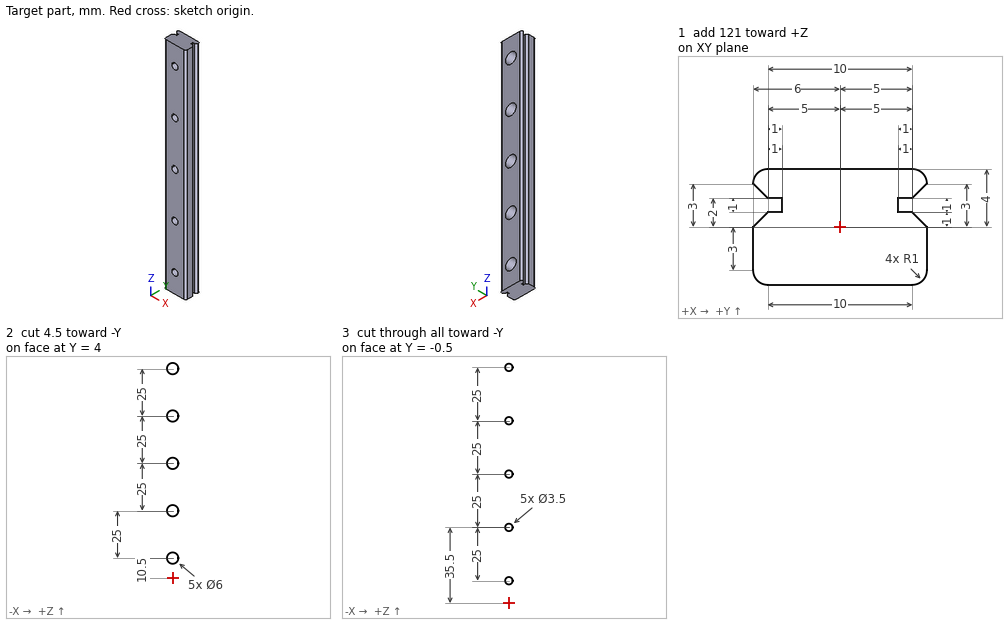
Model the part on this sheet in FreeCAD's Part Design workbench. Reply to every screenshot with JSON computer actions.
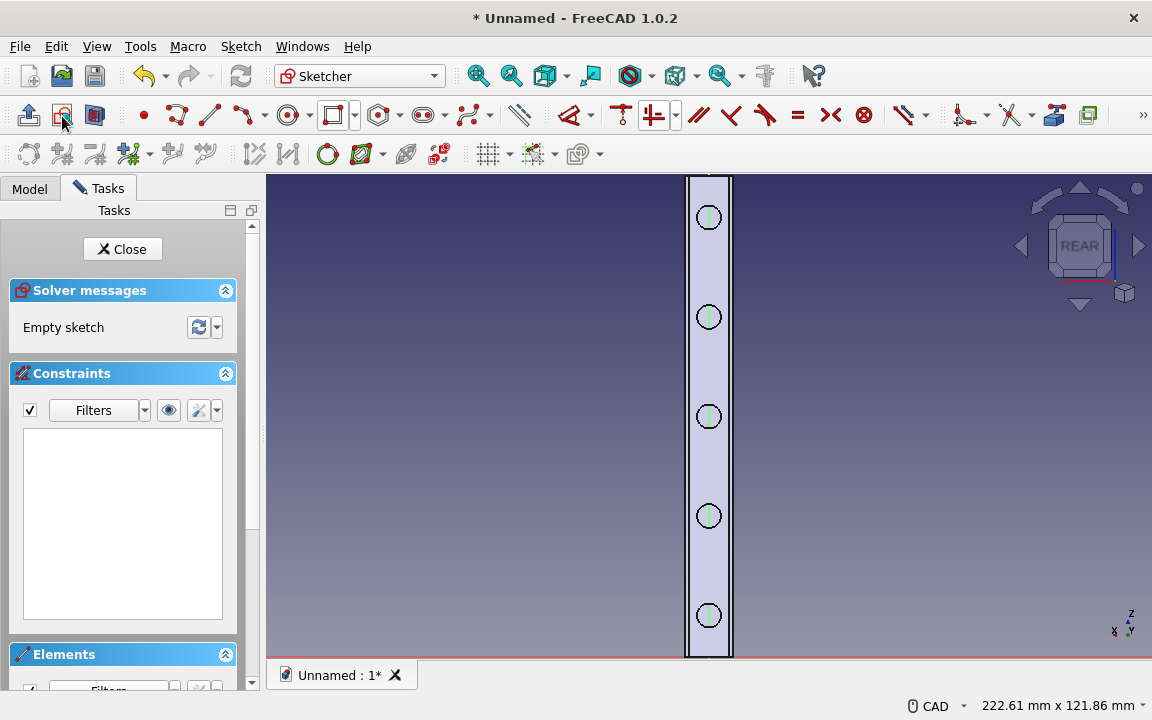
{"action": "scroll", "coordinate": [501, 381], "scroll_direction": "down", "scroll_amount": 2}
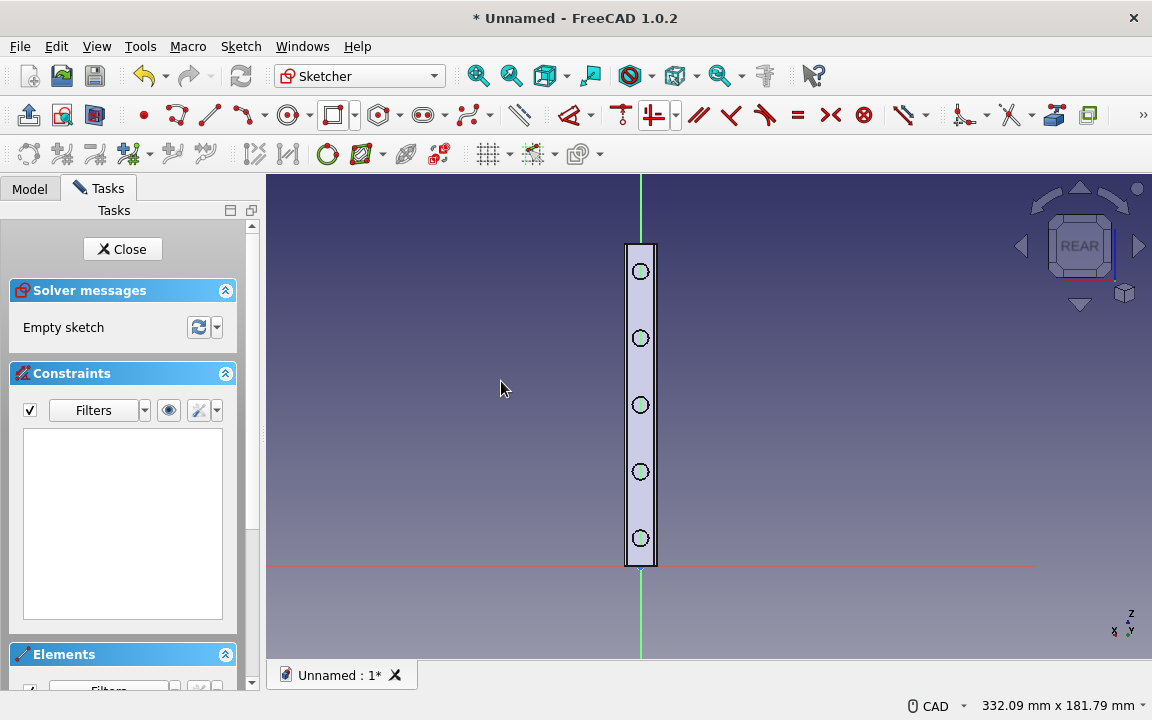
{"action": "left_click", "coordinate": [288, 116]}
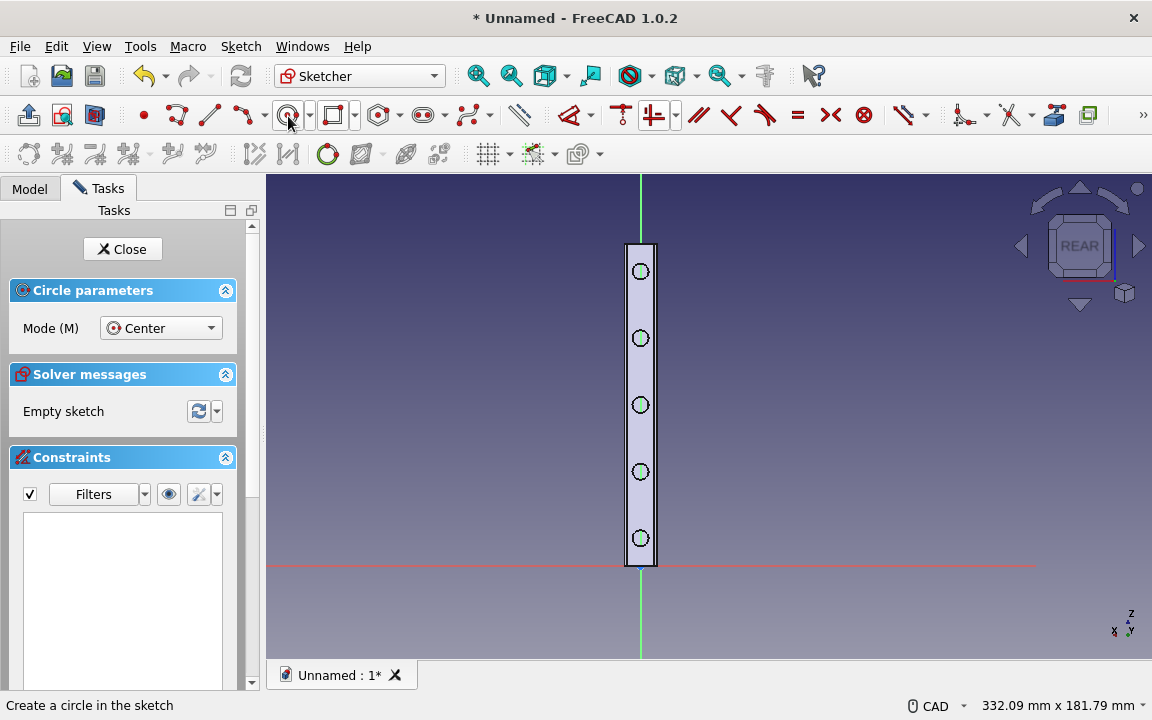
{"action": "scroll", "coordinate": [641, 472], "scroll_direction": "up", "scroll_amount": 8}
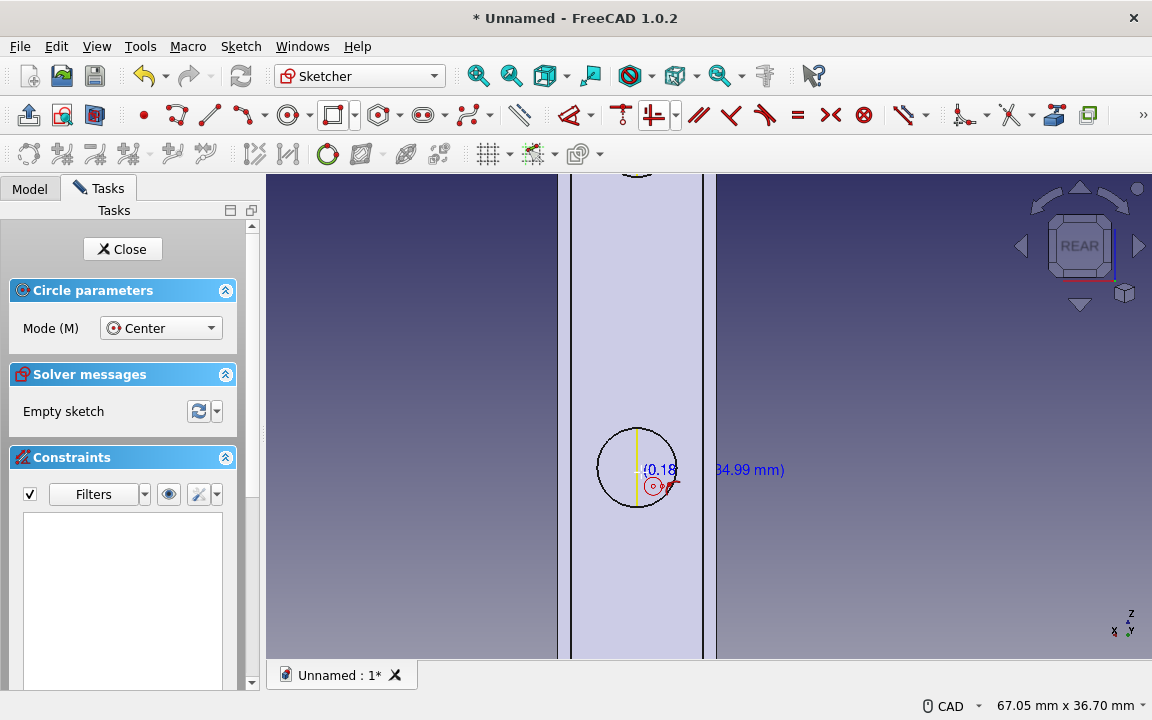
{"action": "scroll", "coordinate": [641, 472], "scroll_direction": "down", "scroll_amount": 8}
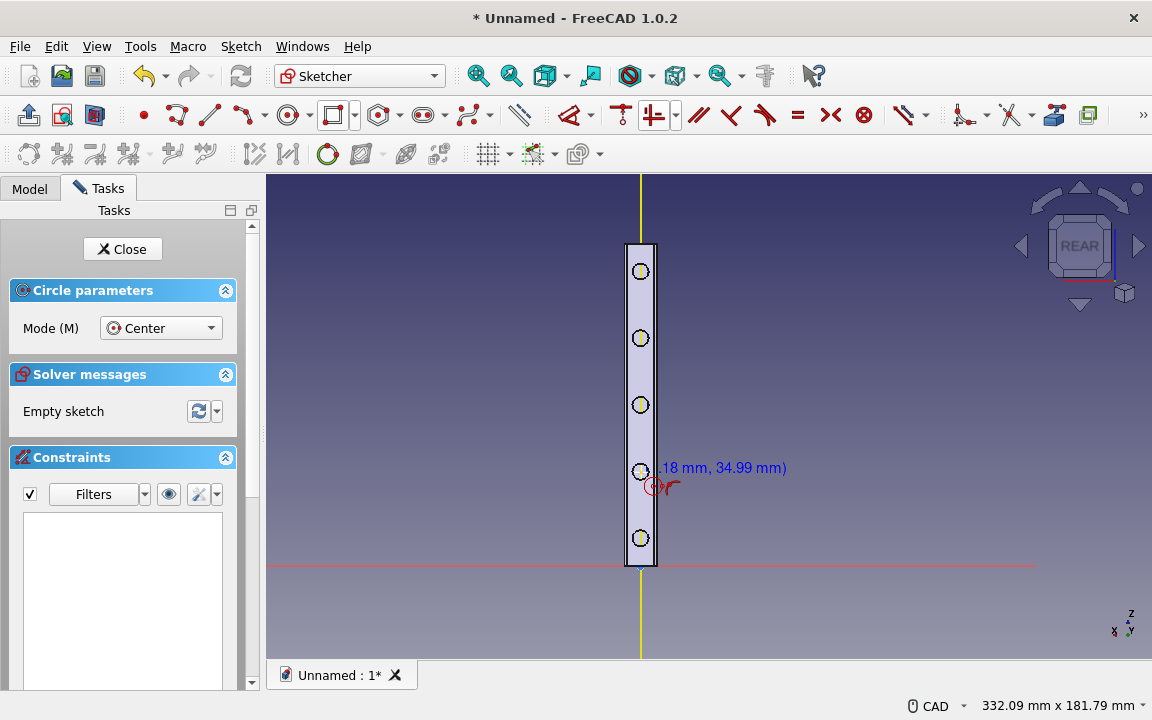
{"action": "left_click", "coordinate": [641, 472]}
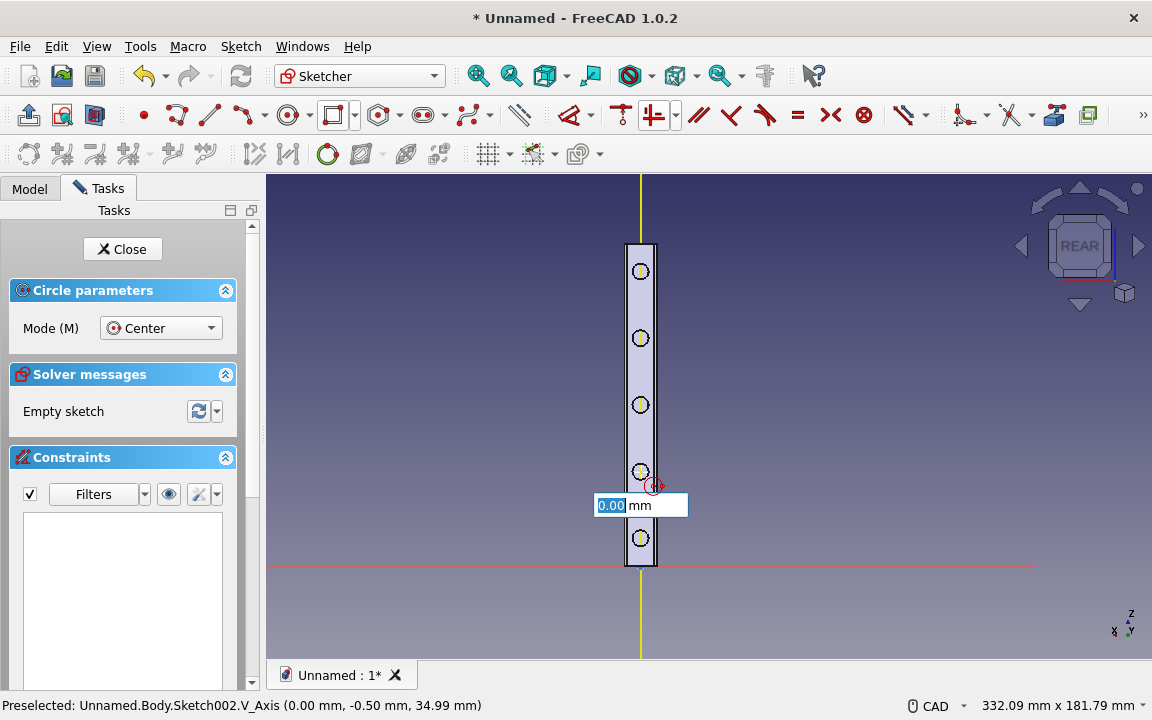
{"action": "scroll", "coordinate": [645, 470], "scroll_direction": "up", "scroll_amount": 7}
{"action": "mouse_move", "coordinate": [643, 468]}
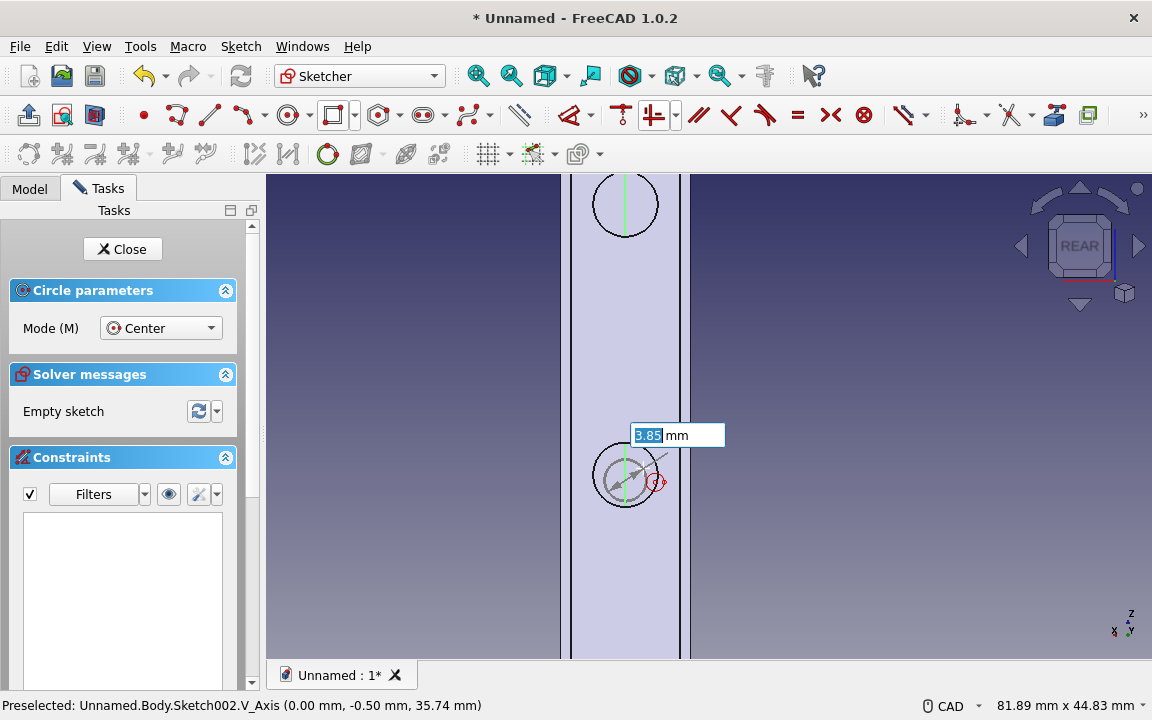
{"action": "type", "text": "3.5"}
{"action": "key", "text": "Return"}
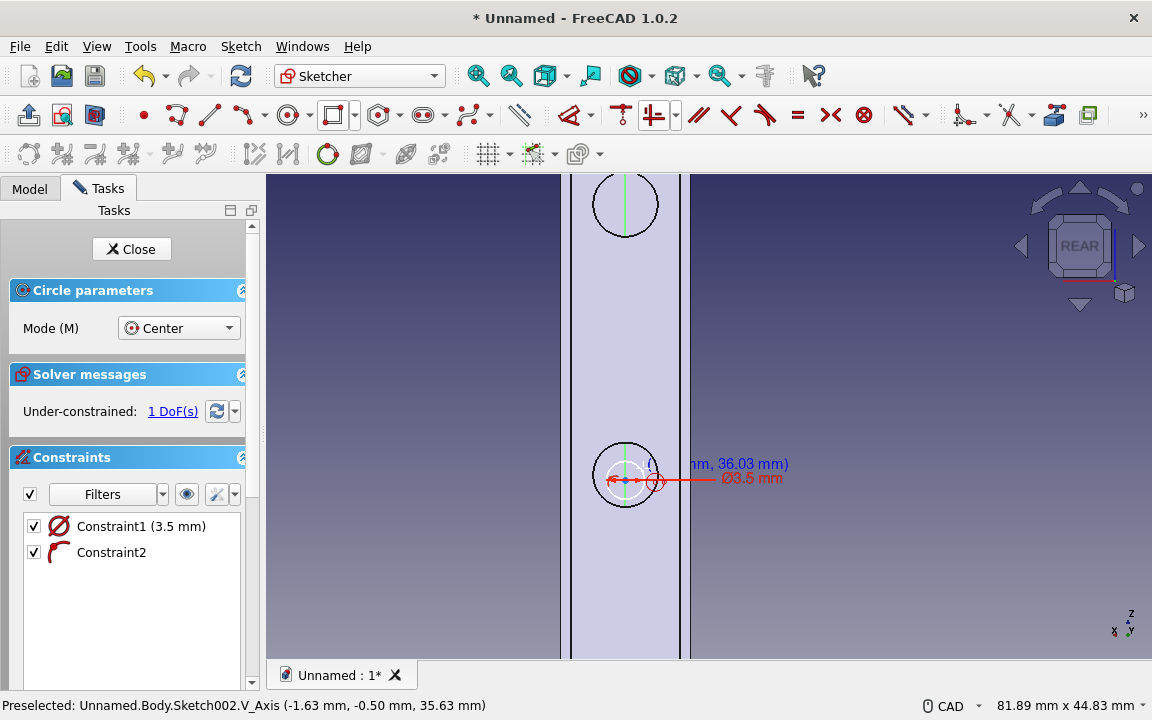
{"action": "scroll", "coordinate": [645, 470], "scroll_direction": "down", "scroll_amount": 7}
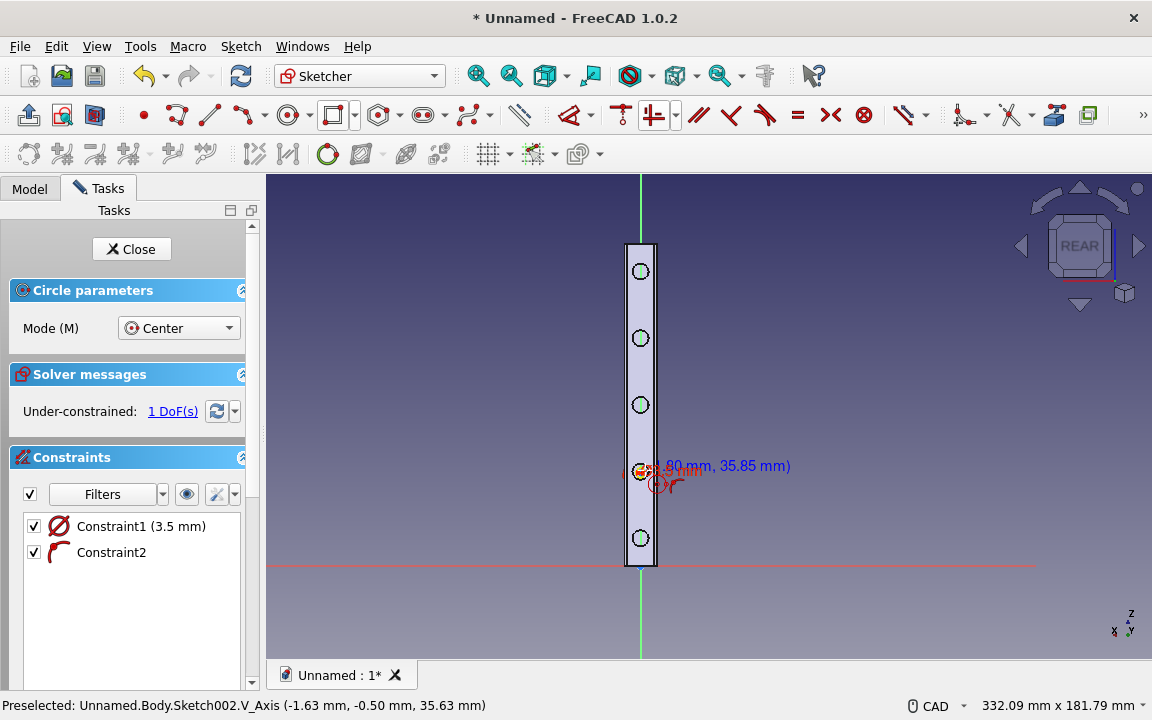
{"action": "scroll", "coordinate": [641, 538], "scroll_direction": "up", "scroll_amount": 8}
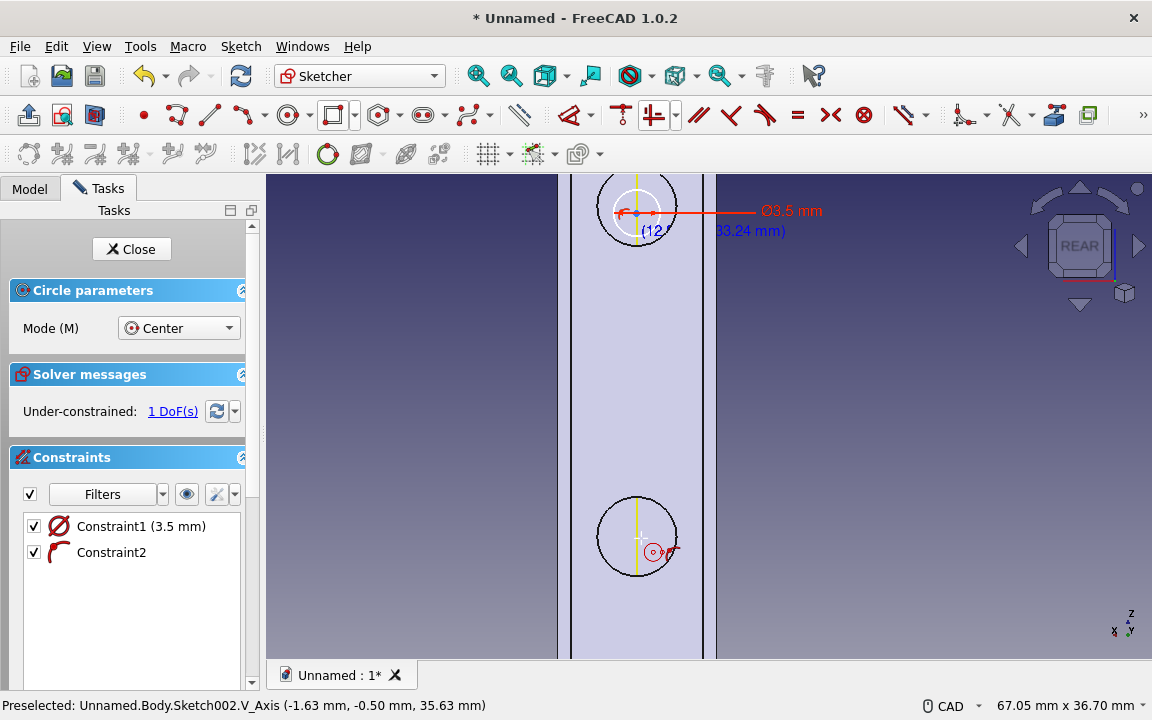
{"action": "scroll", "coordinate": [641, 539], "scroll_direction": "down", "scroll_amount": 8}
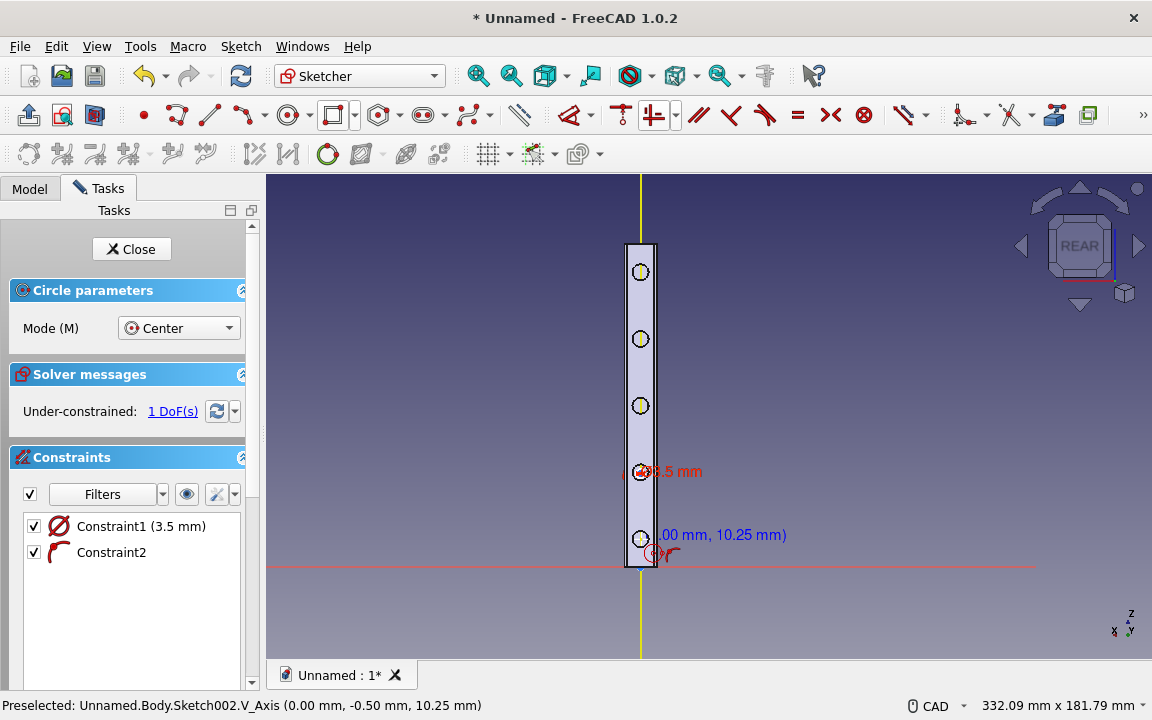
{"action": "left_click", "coordinate": [641, 539]}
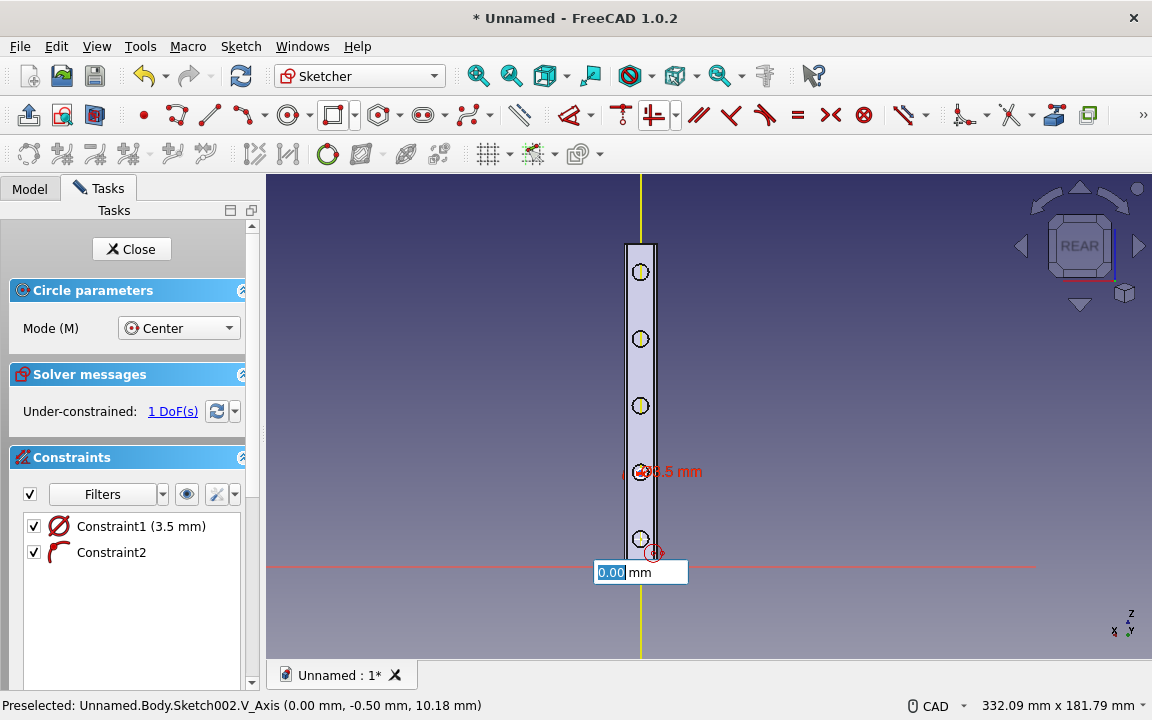
{"action": "scroll", "coordinate": [645, 538], "scroll_direction": "up", "scroll_amount": 7}
{"action": "mouse_move", "coordinate": [643, 534]}